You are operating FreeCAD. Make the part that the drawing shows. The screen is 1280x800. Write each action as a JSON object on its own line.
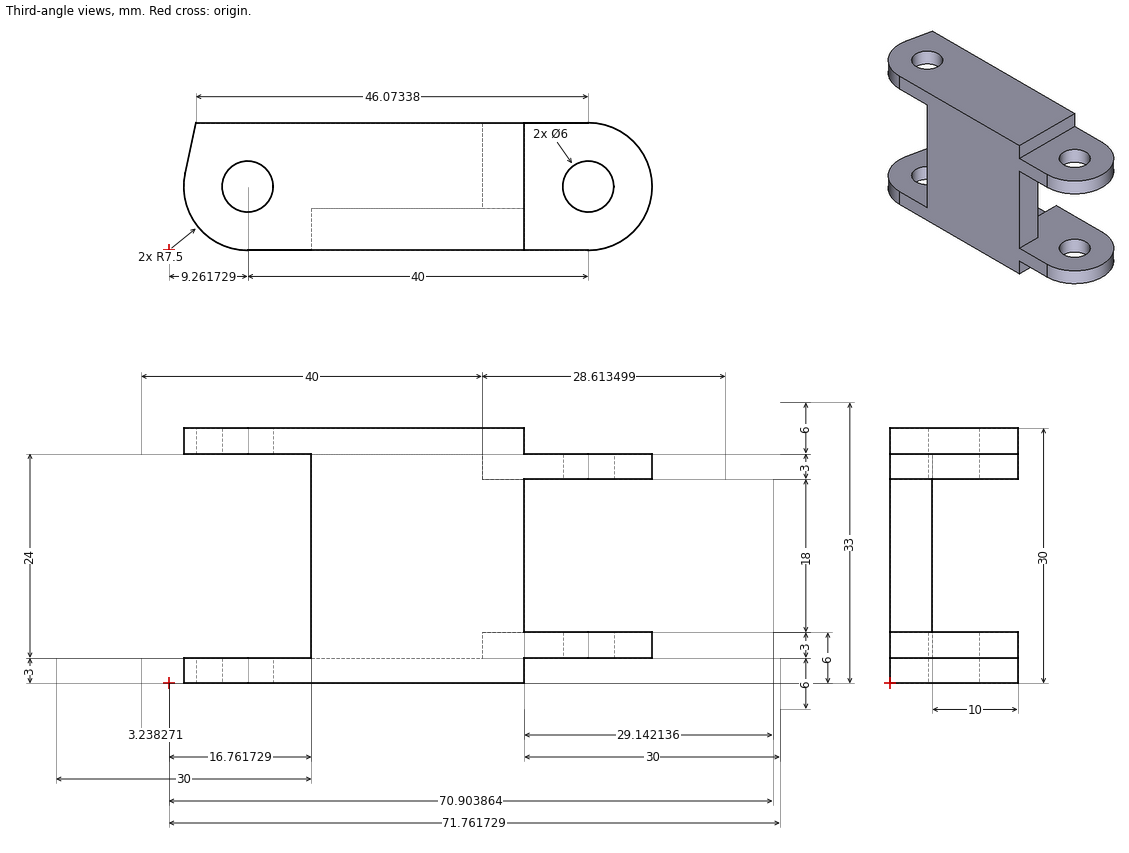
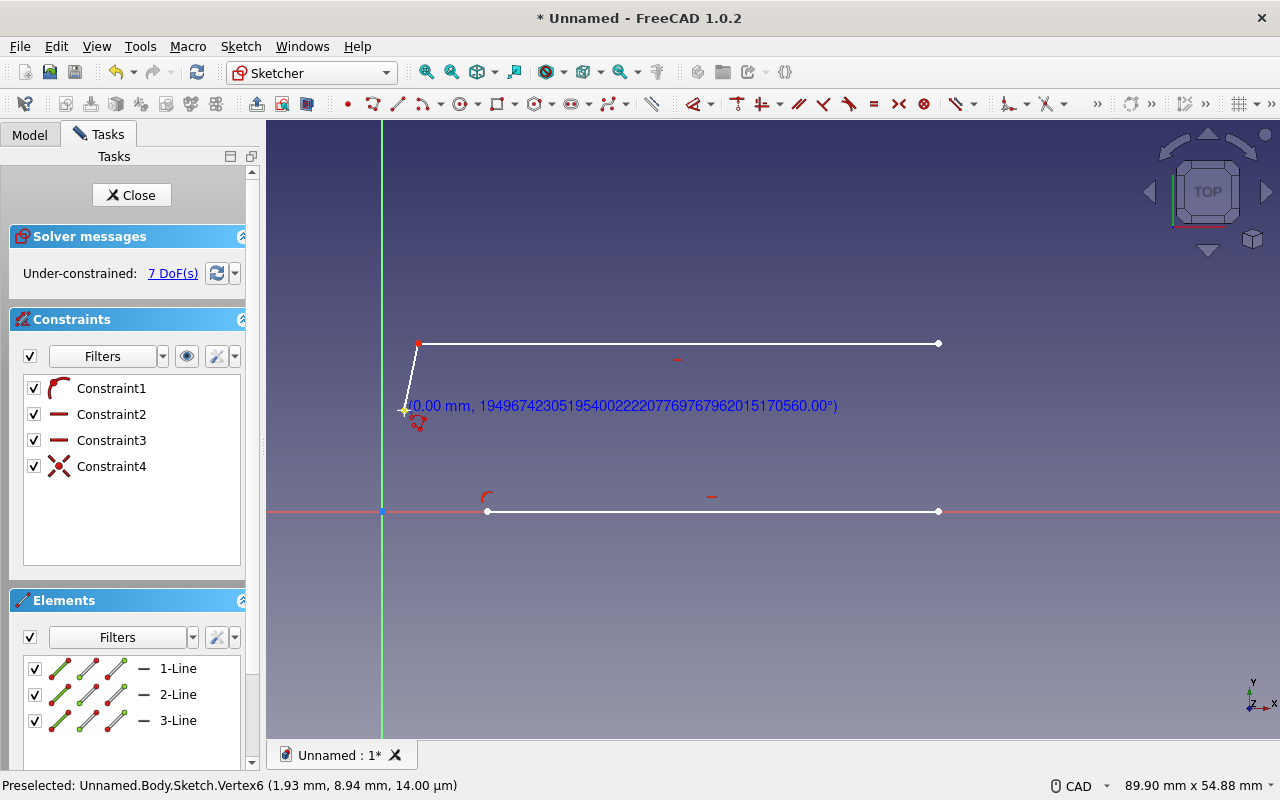
{"action": "key", "text": "g 3 a"}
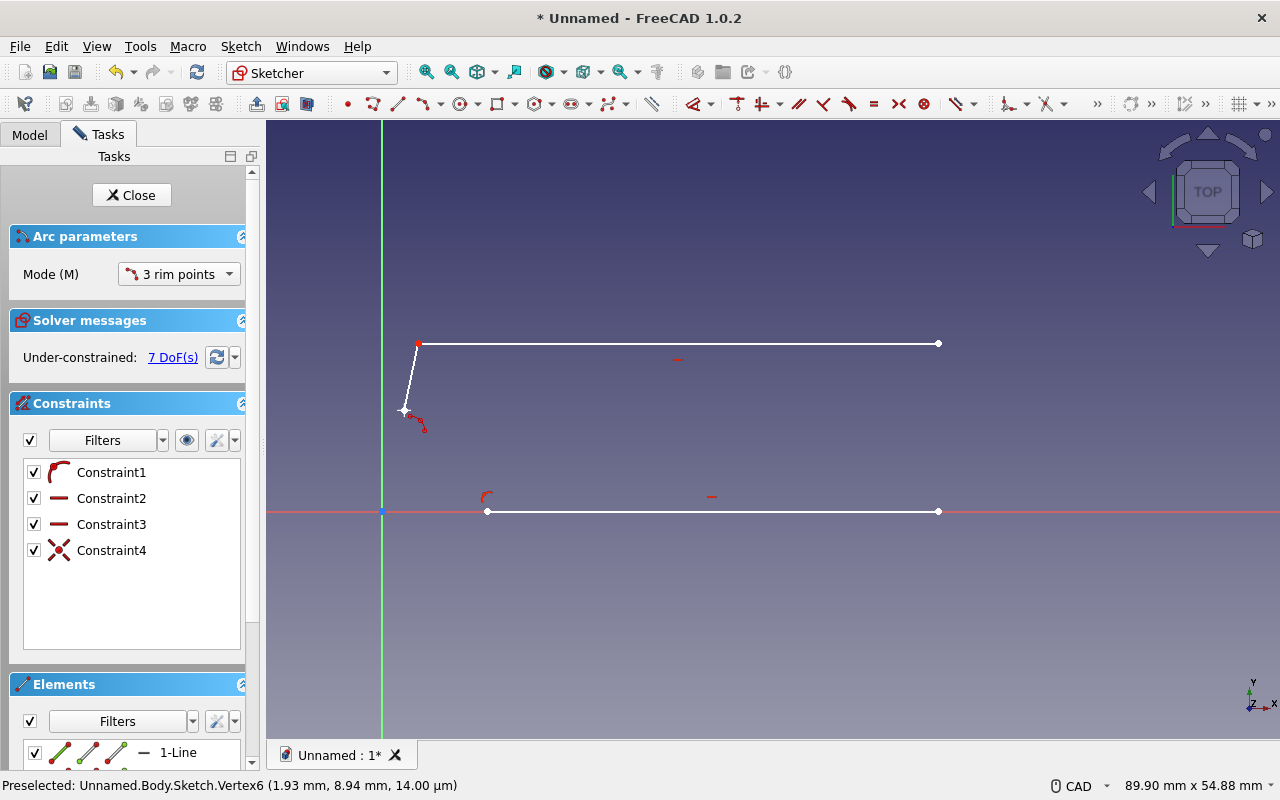
{"action": "left_click", "coordinate": [938, 512]}
{"action": "left_click", "coordinate": [938, 344]}
{"action": "left_click", "coordinate": [1022, 427]}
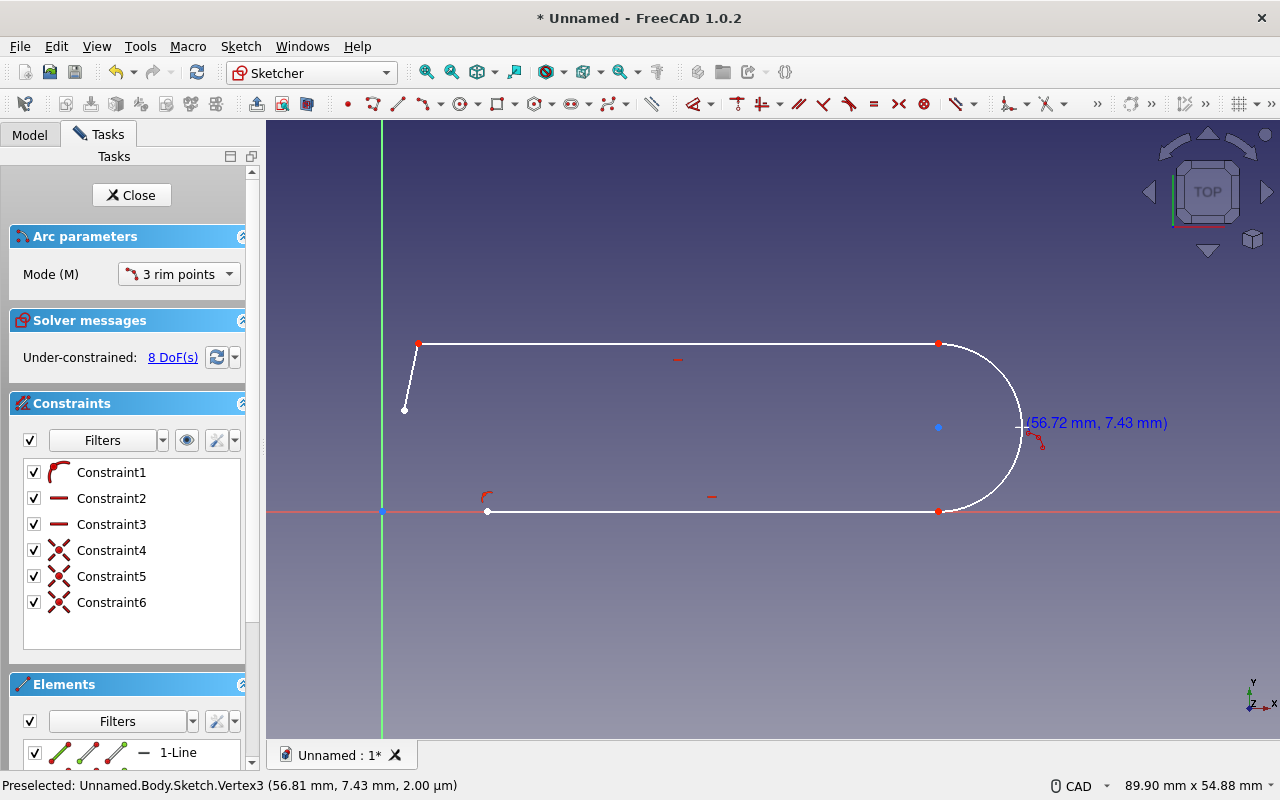
{"action": "left_click", "coordinate": [404, 411]}
{"action": "left_click", "coordinate": [487, 512]}
{"action": "left_click", "coordinate": [421, 480]}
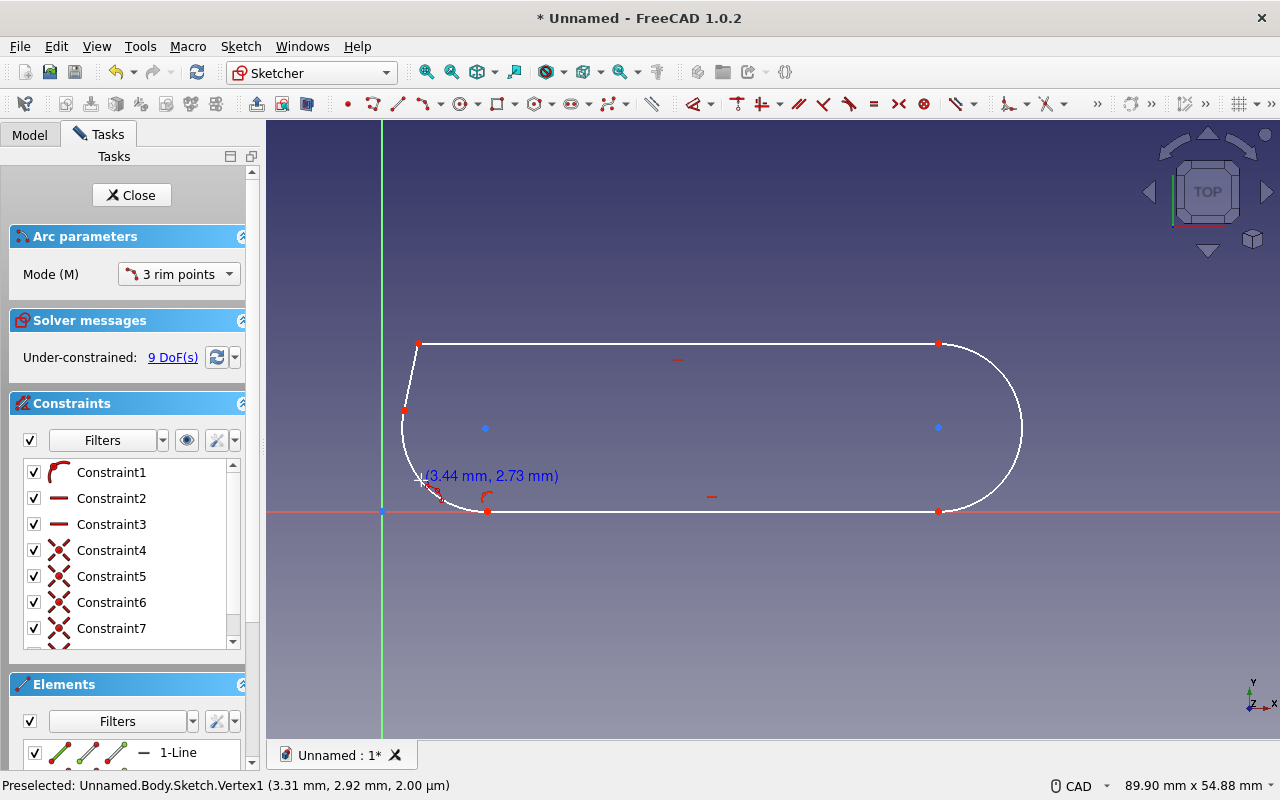
{"action": "left_click", "coordinate": [460, 104]}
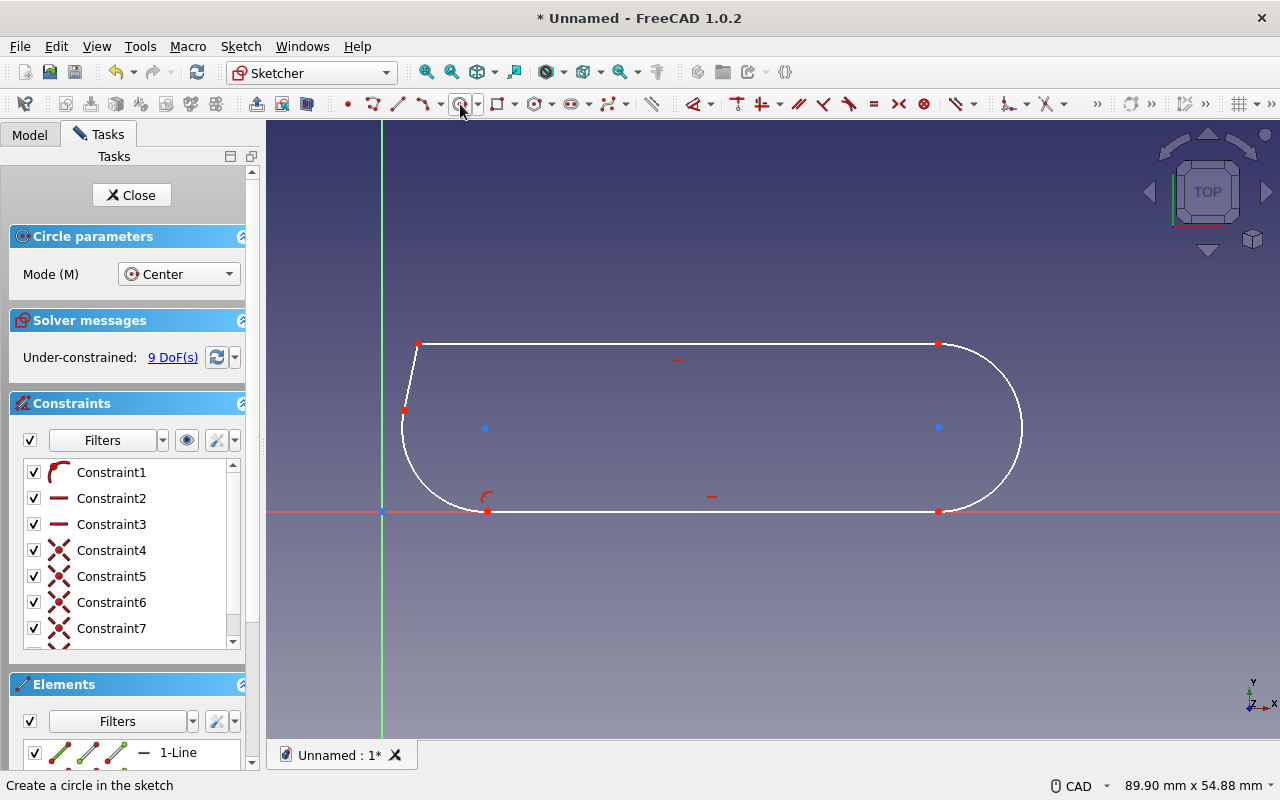
{"action": "left_click", "coordinate": [938, 427]}
{"action": "left_click", "coordinate": [962, 403]}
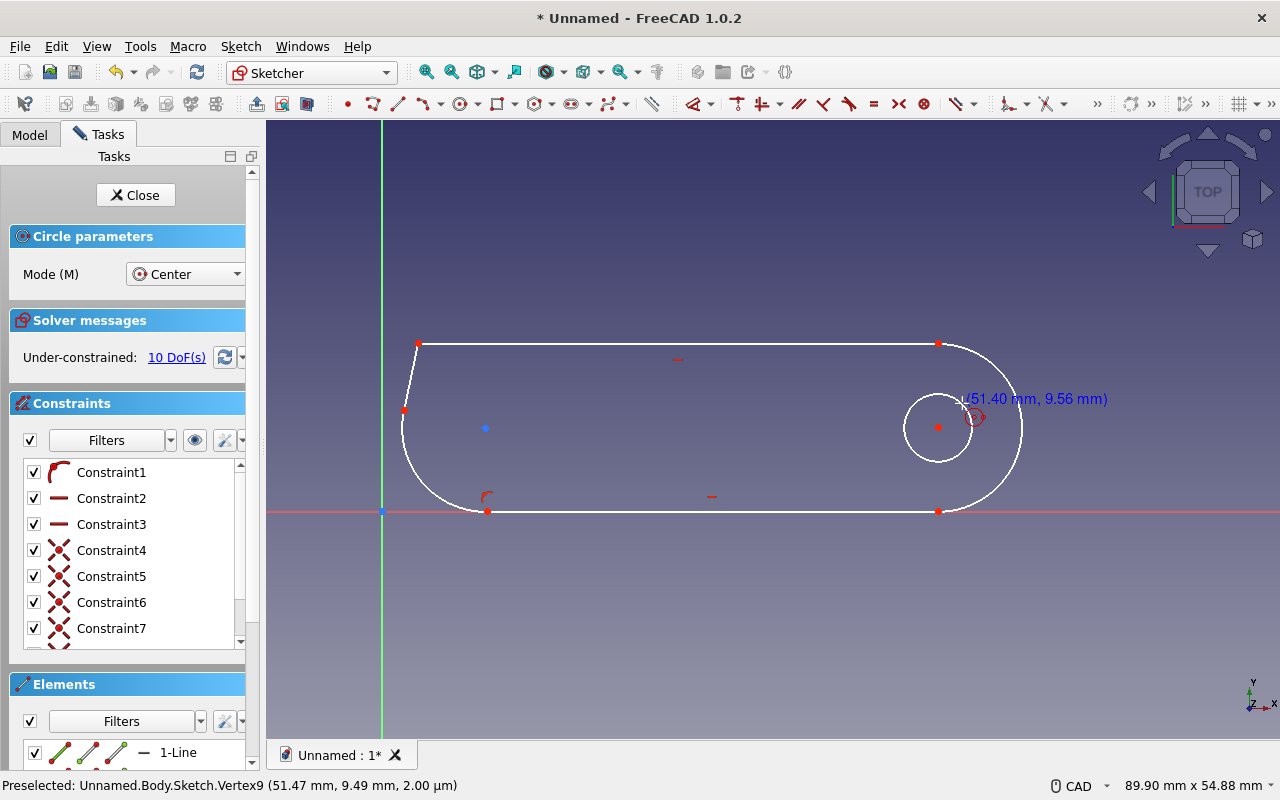
{"action": "left_click", "coordinate": [487, 427]}
{"action": "left_click", "coordinate": [511, 403]}
{"action": "key", "text": "Escape"}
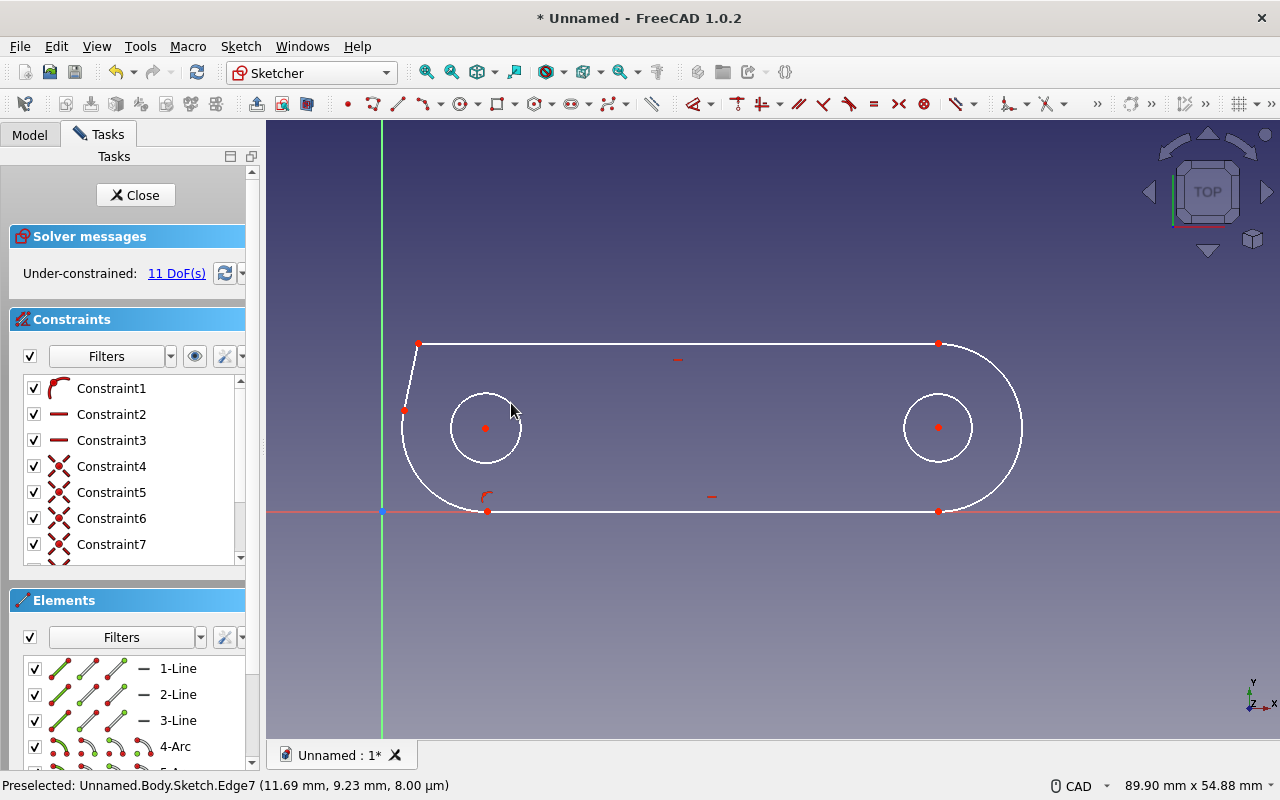
{"action": "left_click", "coordinate": [622, 512]}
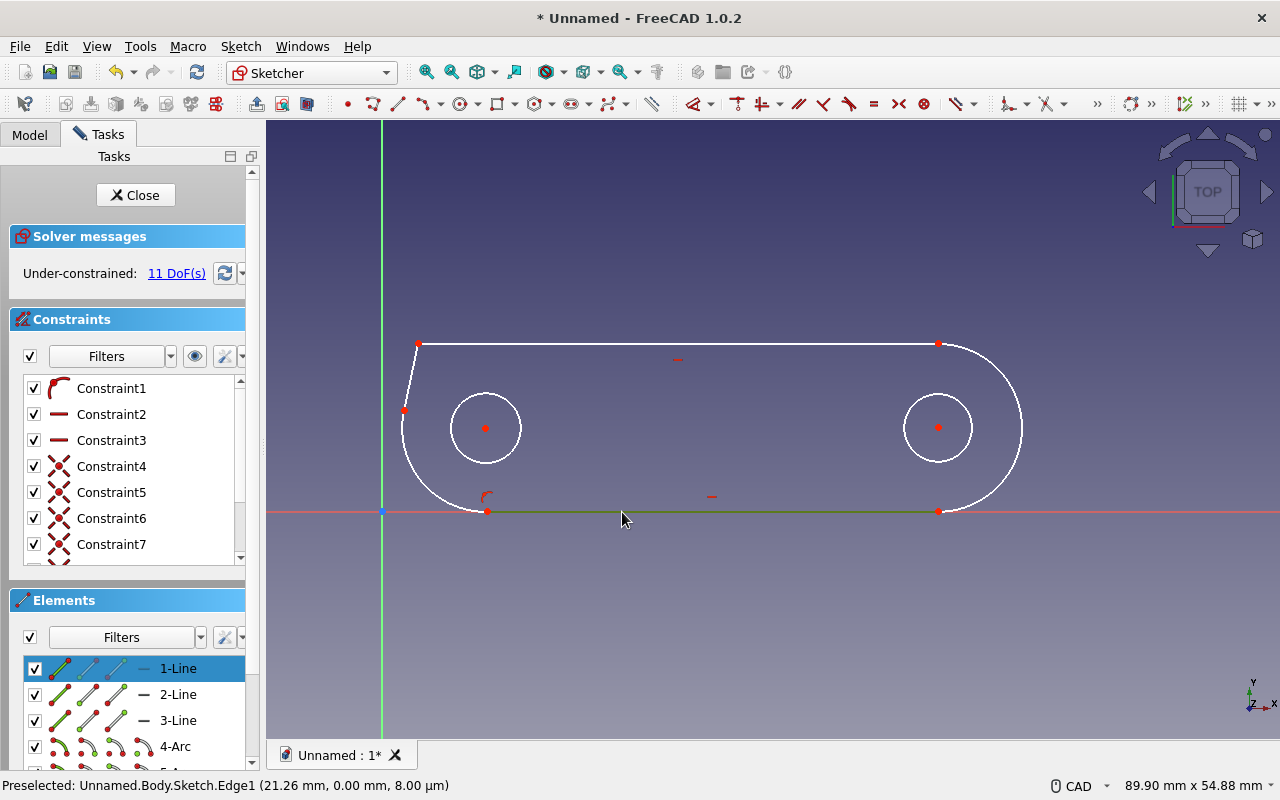
{"action": "left_click", "coordinate": [1006, 477]}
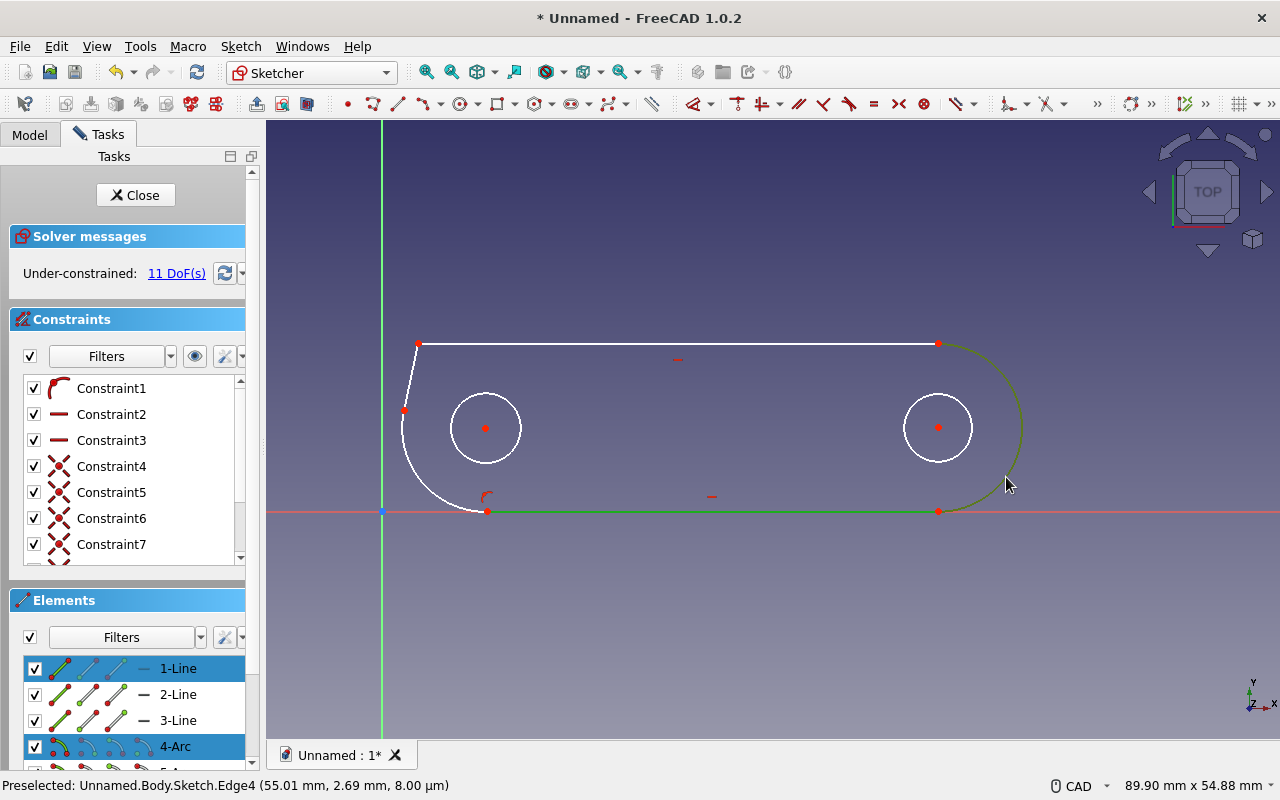
{"action": "left_click", "coordinate": [849, 104]}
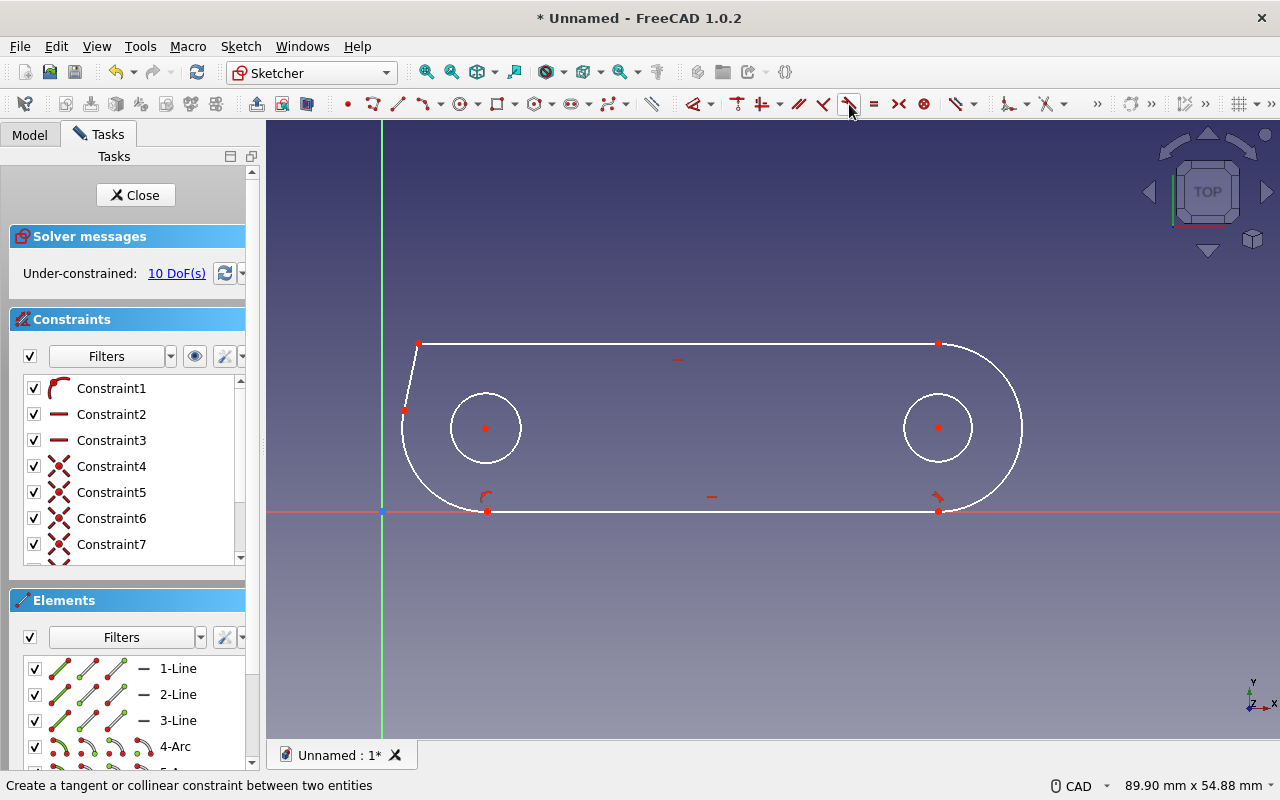
{"action": "left_click", "coordinate": [622, 512]}